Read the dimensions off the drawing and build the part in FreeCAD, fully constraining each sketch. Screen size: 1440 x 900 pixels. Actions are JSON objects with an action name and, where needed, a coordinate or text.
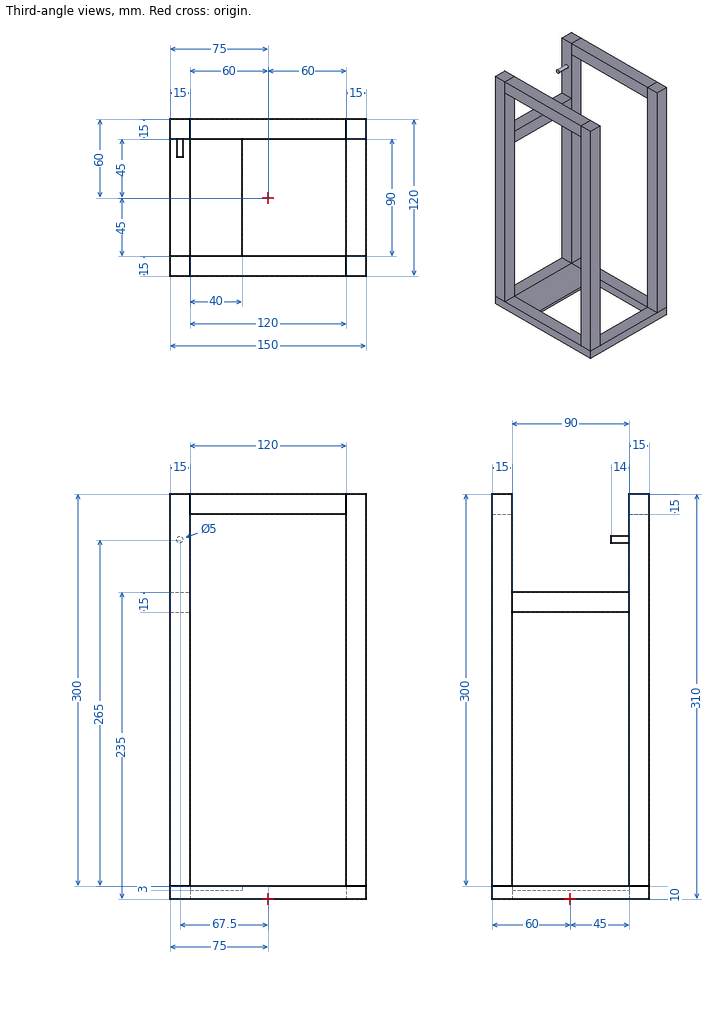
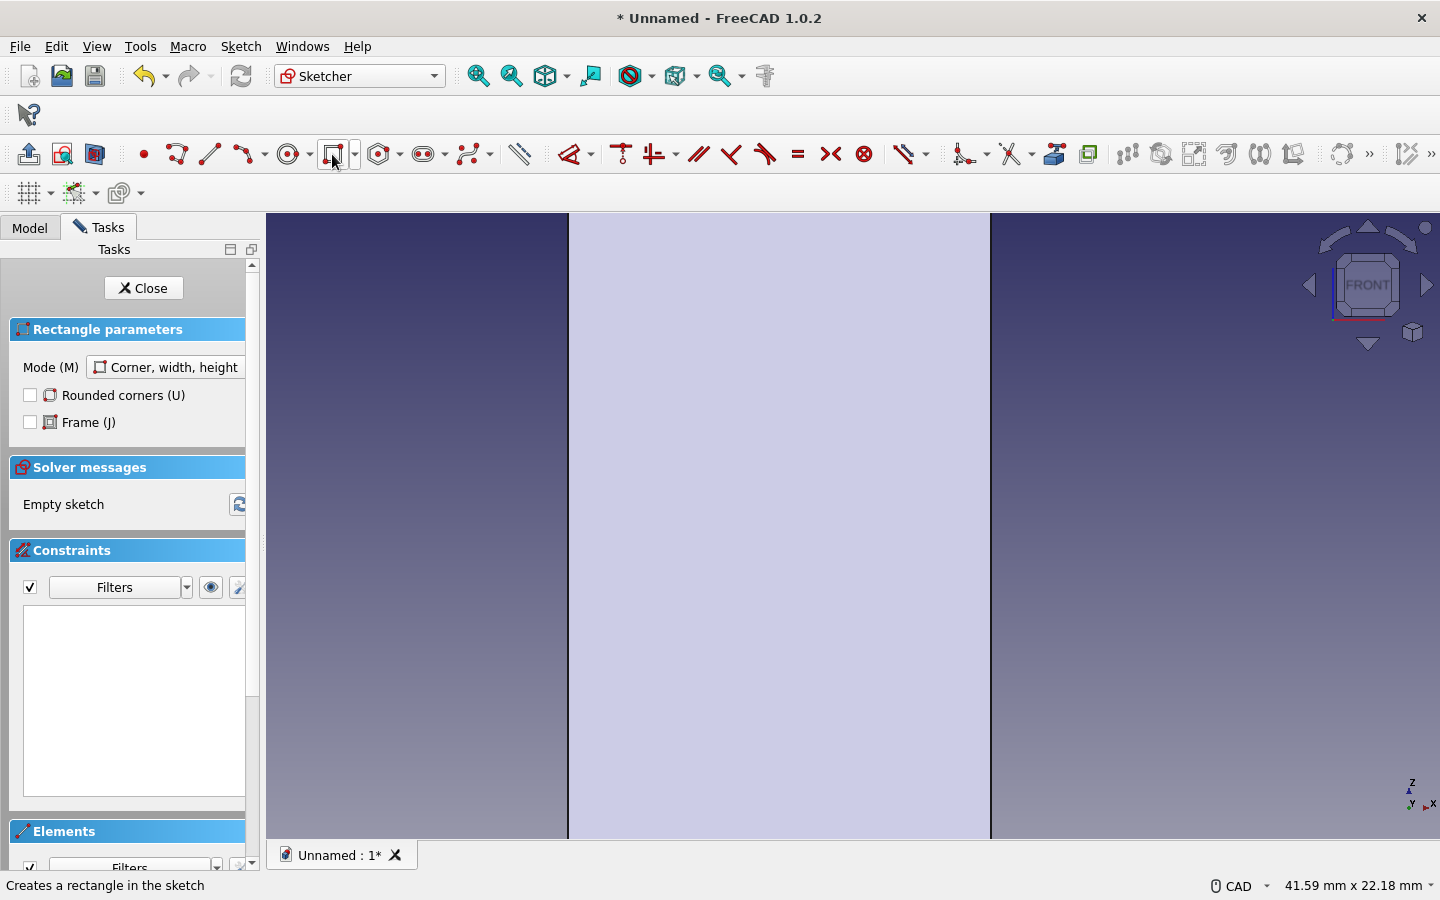
{"action": "left_click", "coordinate": [568, 317]}
{"action": "left_click", "coordinate": [991, 741]}
{"action": "key", "text": "Escape"}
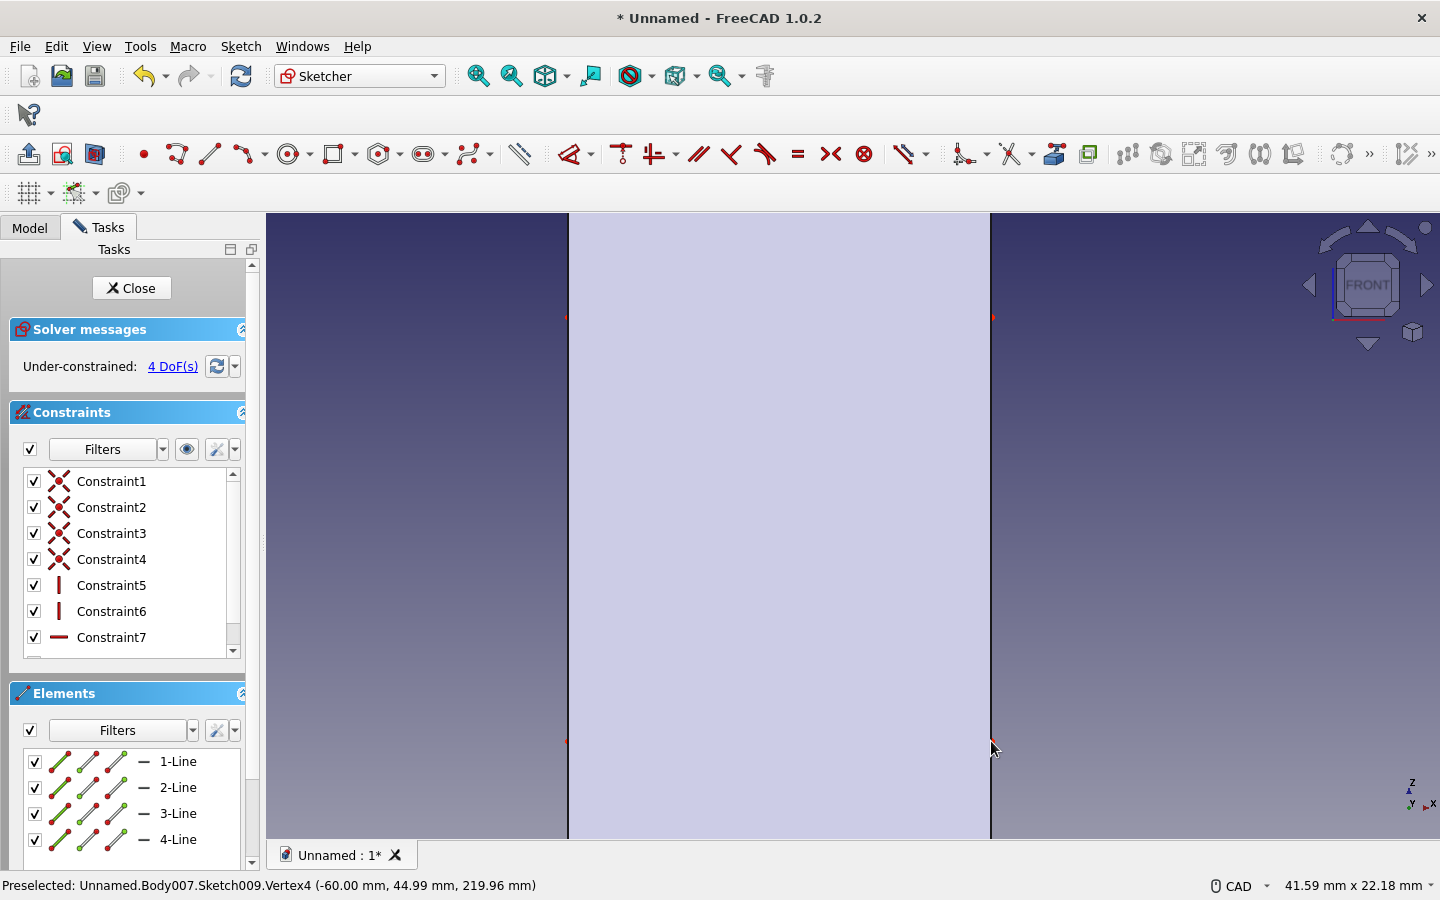
{"action": "left_click", "coordinate": [568, 154]}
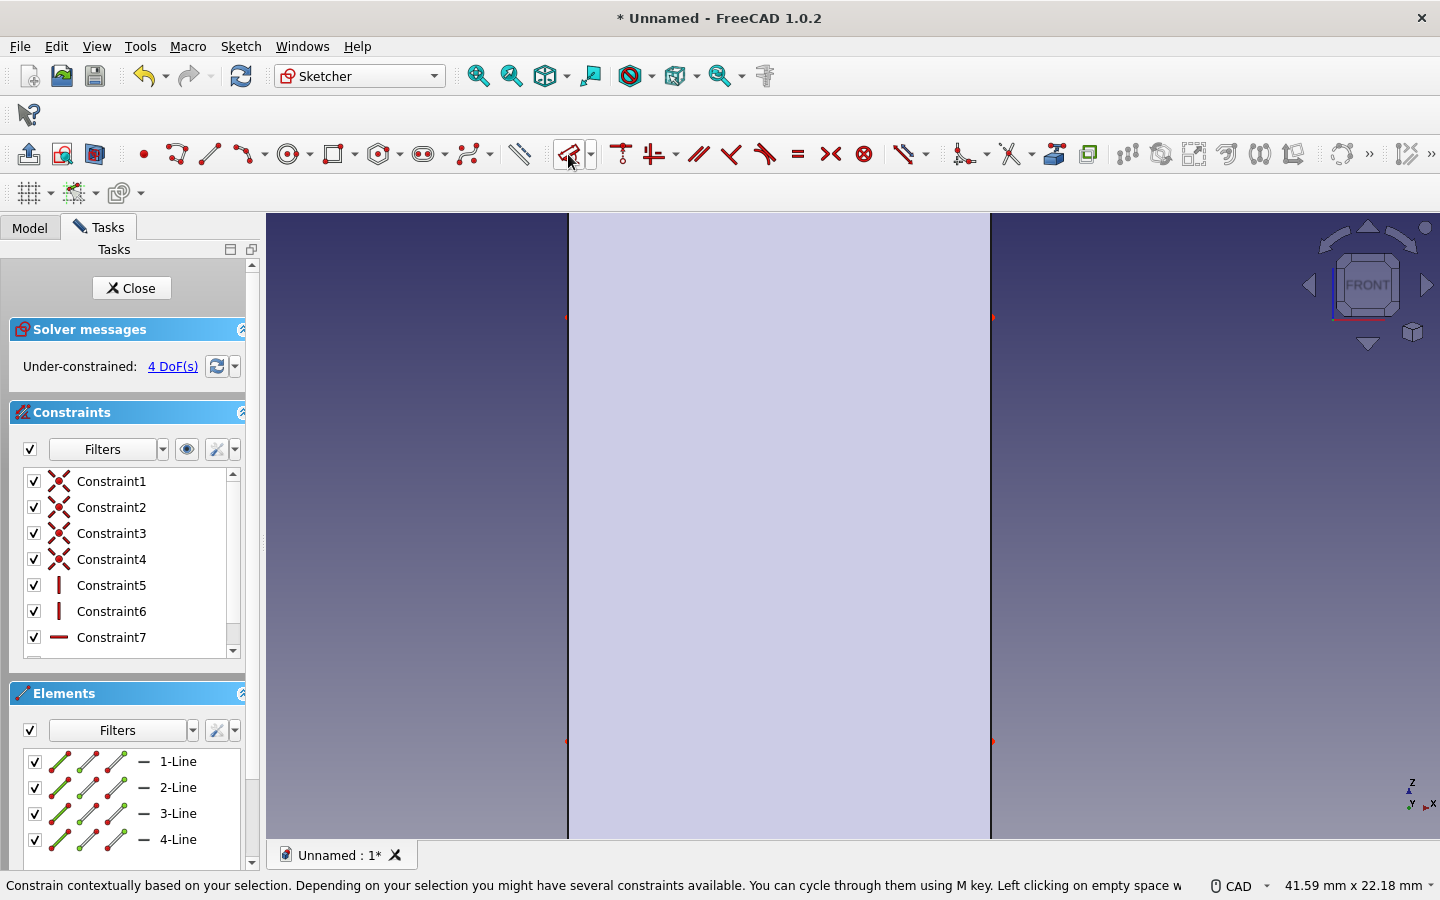
{"action": "left_click", "coordinate": [568, 445]}
{"action": "left_click", "coordinate": [534, 530]}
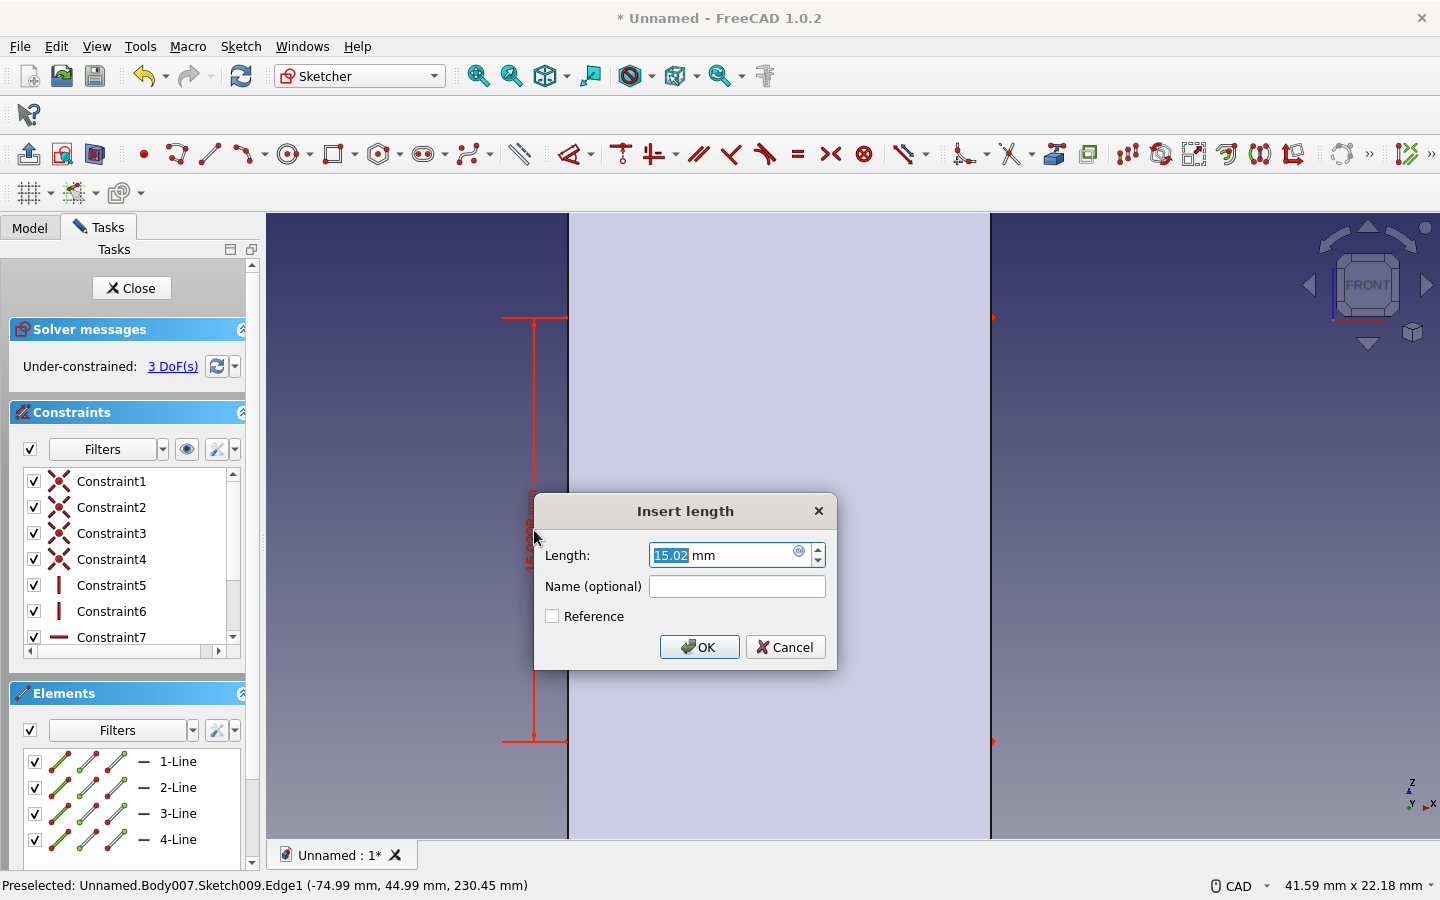
{"action": "type", "text": "15"}
{"action": "key", "text": "Return"}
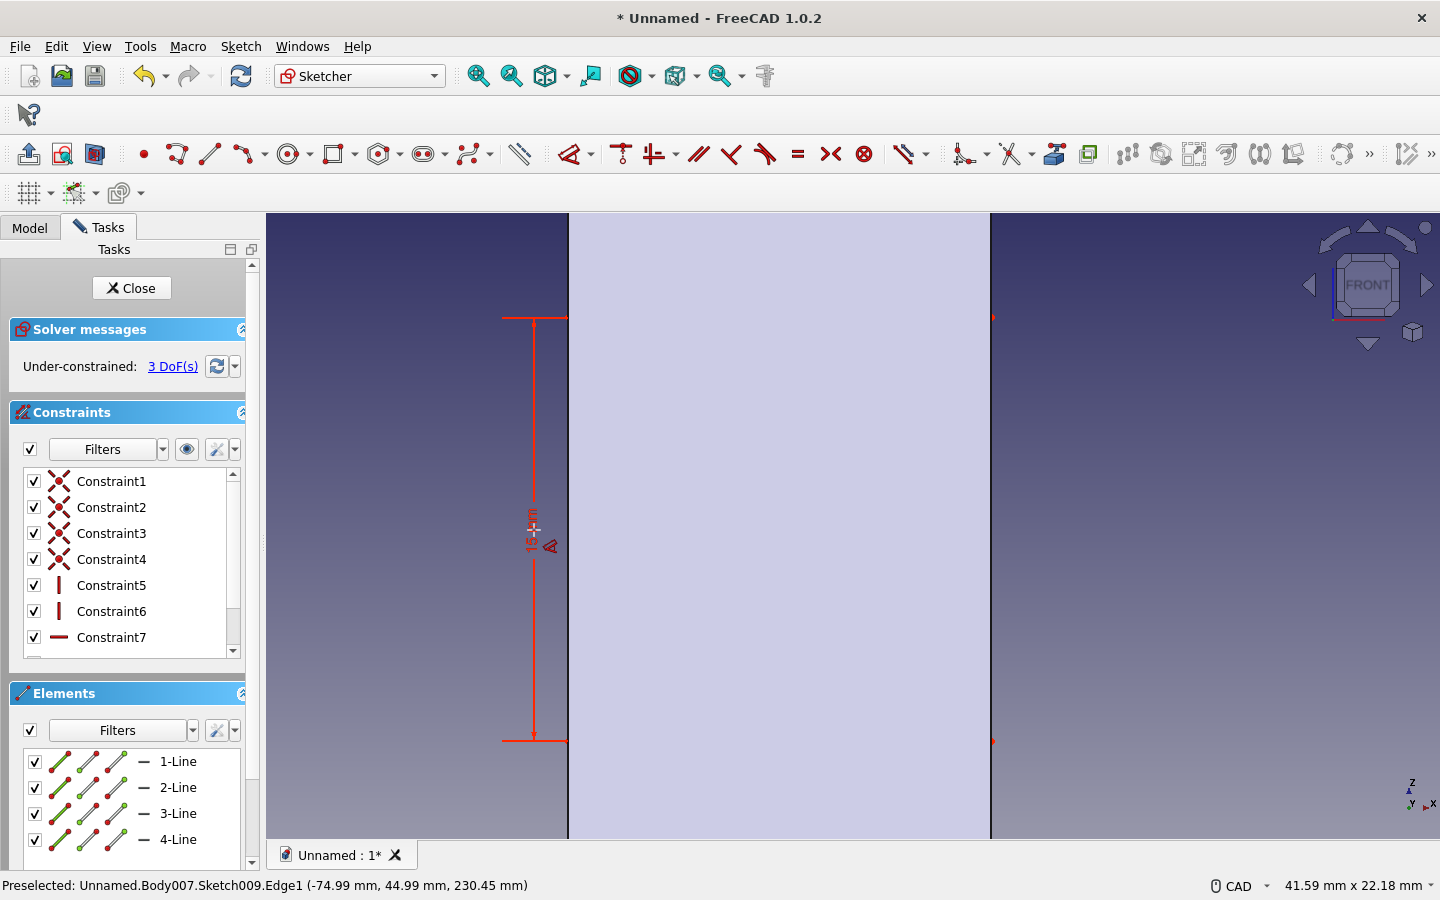
{"action": "left_click", "coordinate": [695, 741]}
{"action": "left_click", "coordinate": [779, 775]}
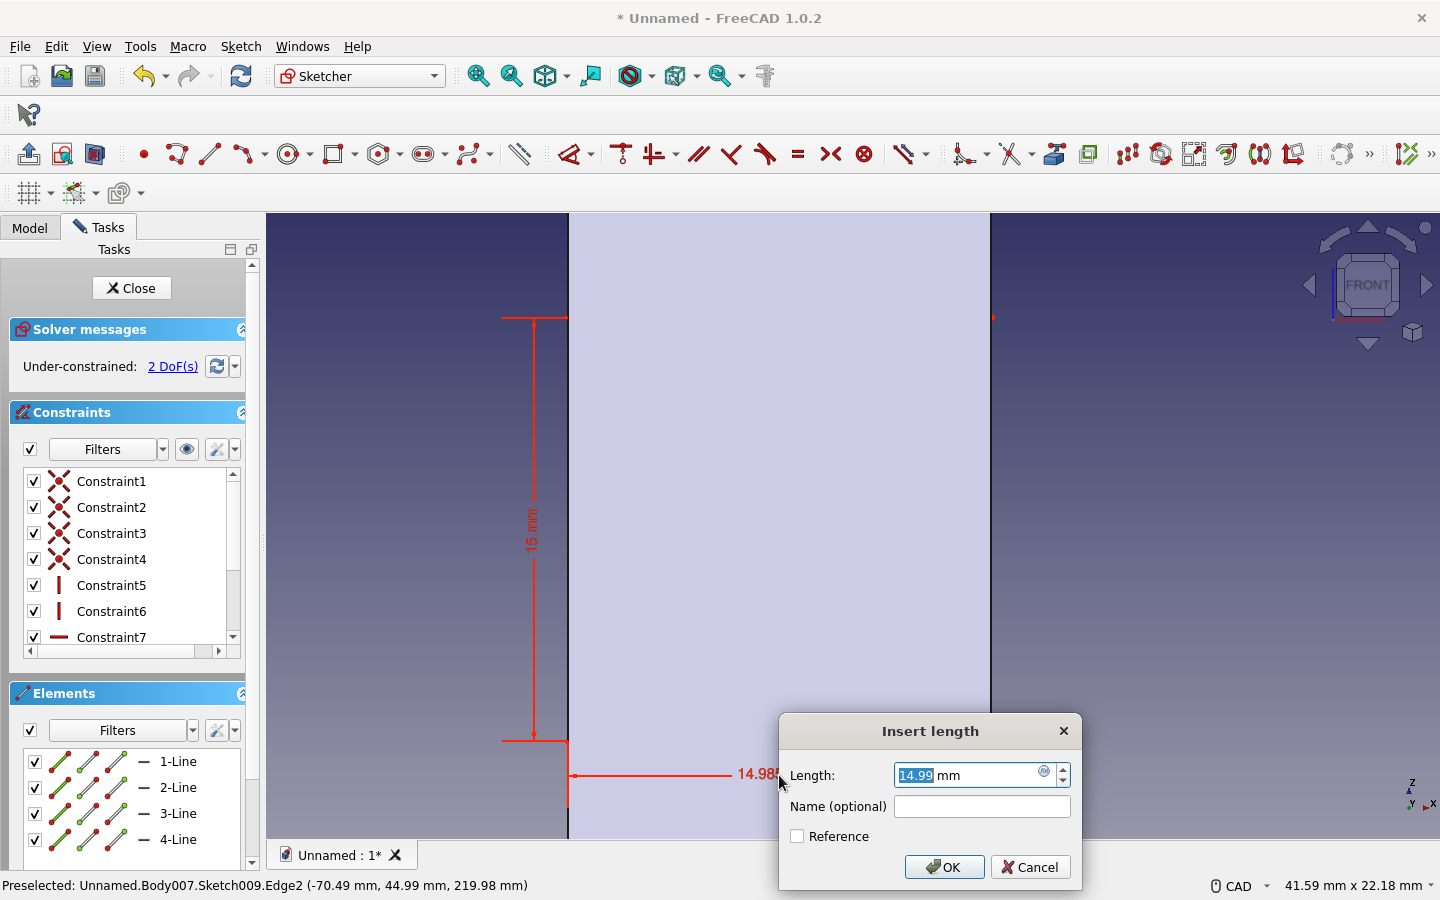
{"action": "type", "text": "15"}
{"action": "key", "text": "Return"}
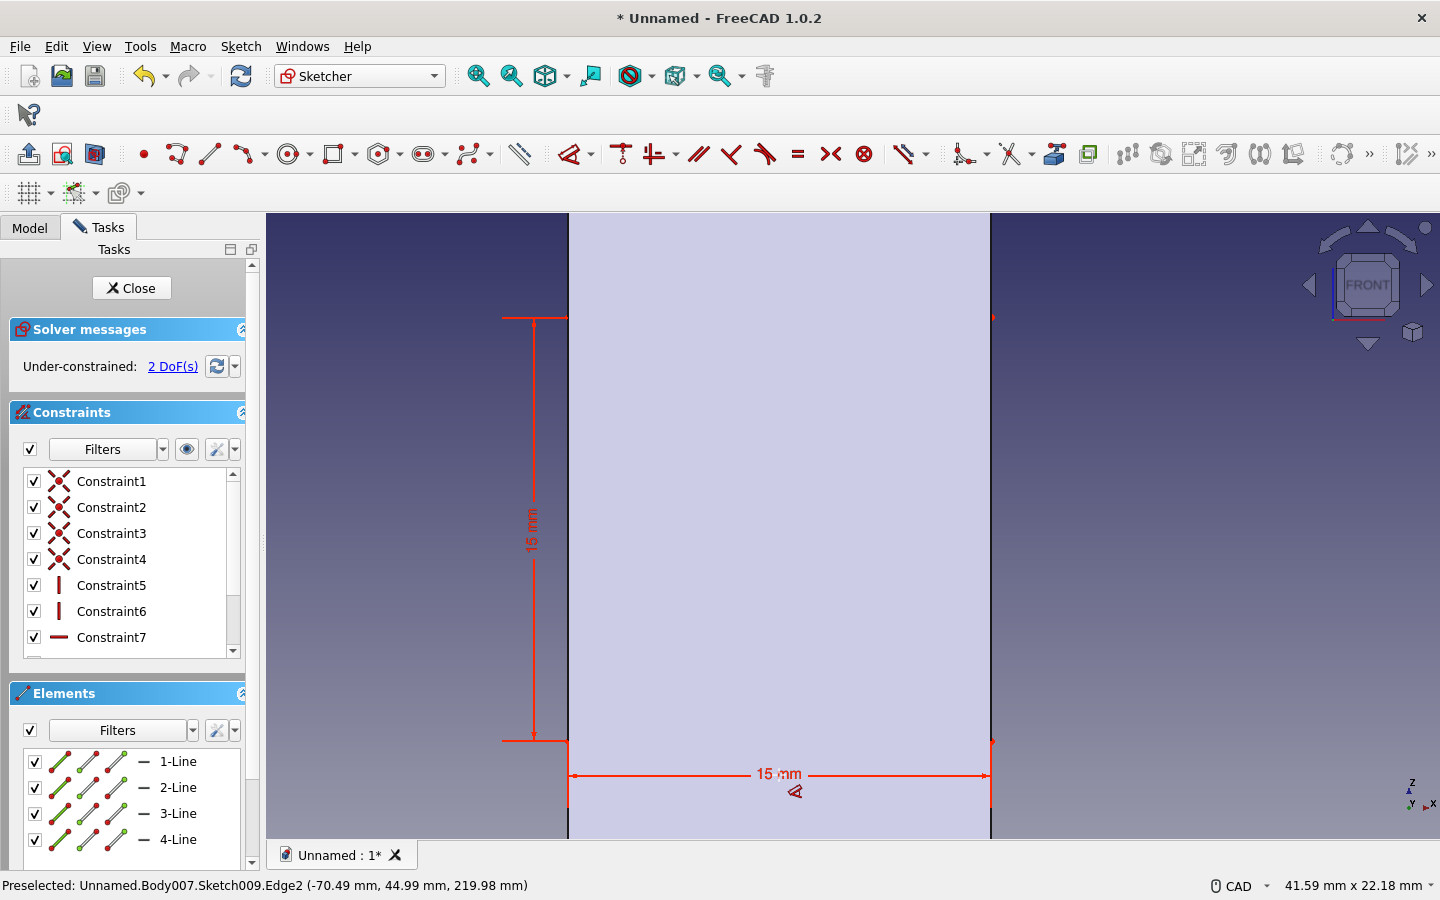
{"action": "left_click", "coordinate": [568, 318]}
{"action": "left_click", "coordinate": [921, 284]}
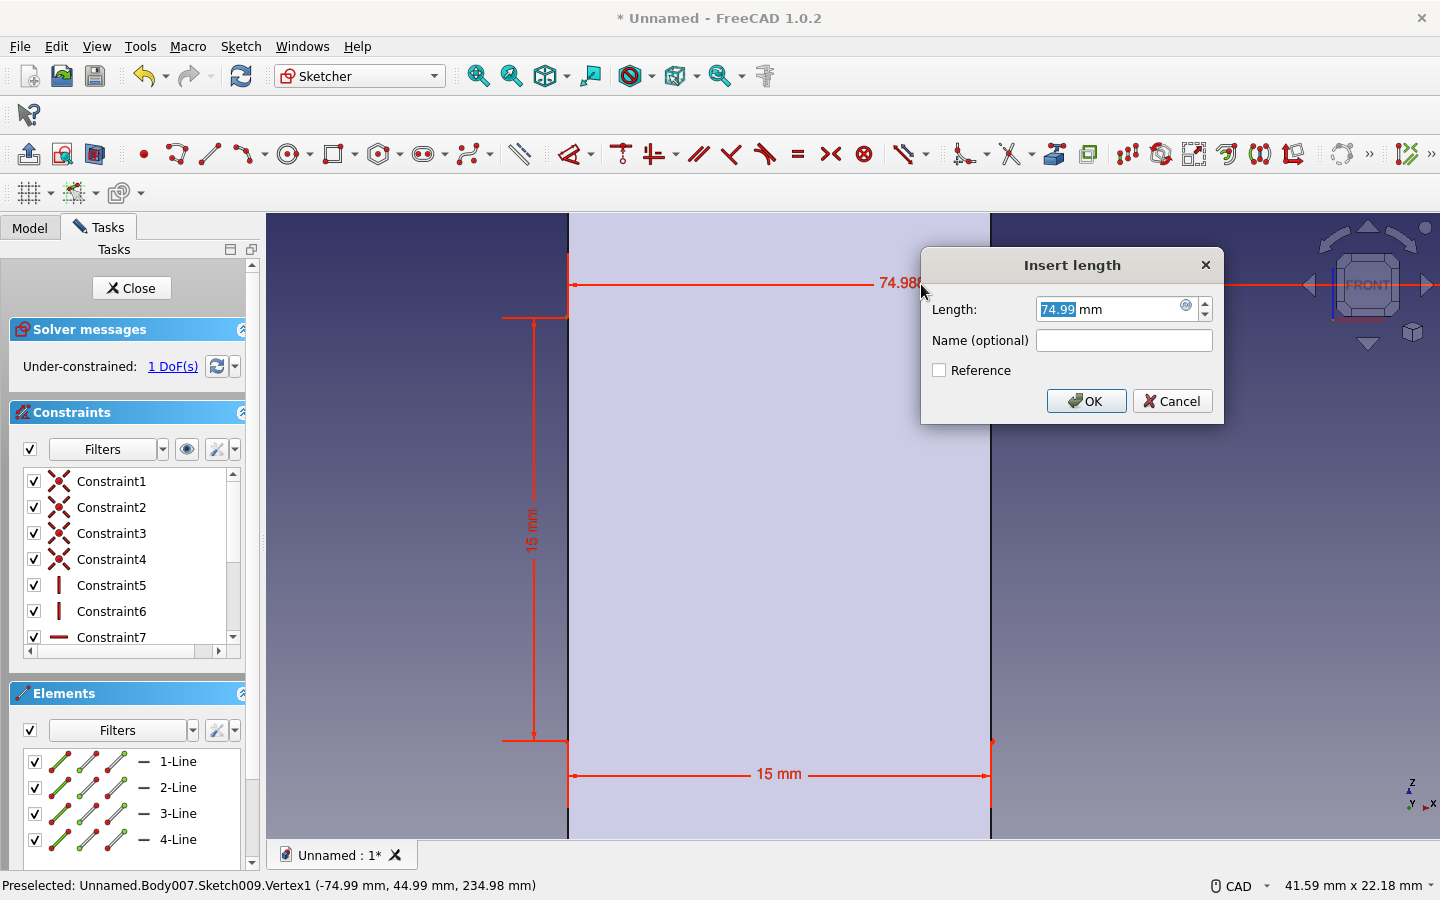
{"action": "type", "text": "75"}
{"action": "key", "text": "Return"}